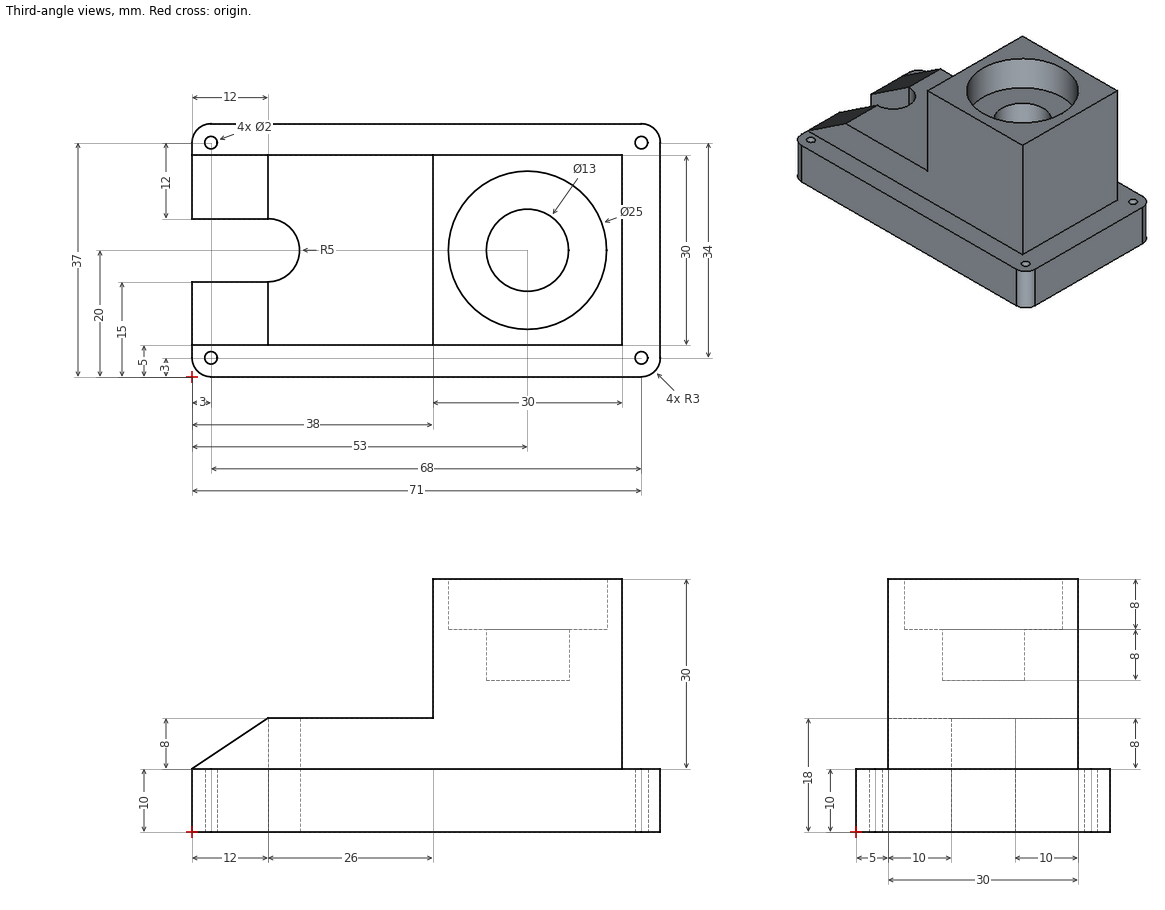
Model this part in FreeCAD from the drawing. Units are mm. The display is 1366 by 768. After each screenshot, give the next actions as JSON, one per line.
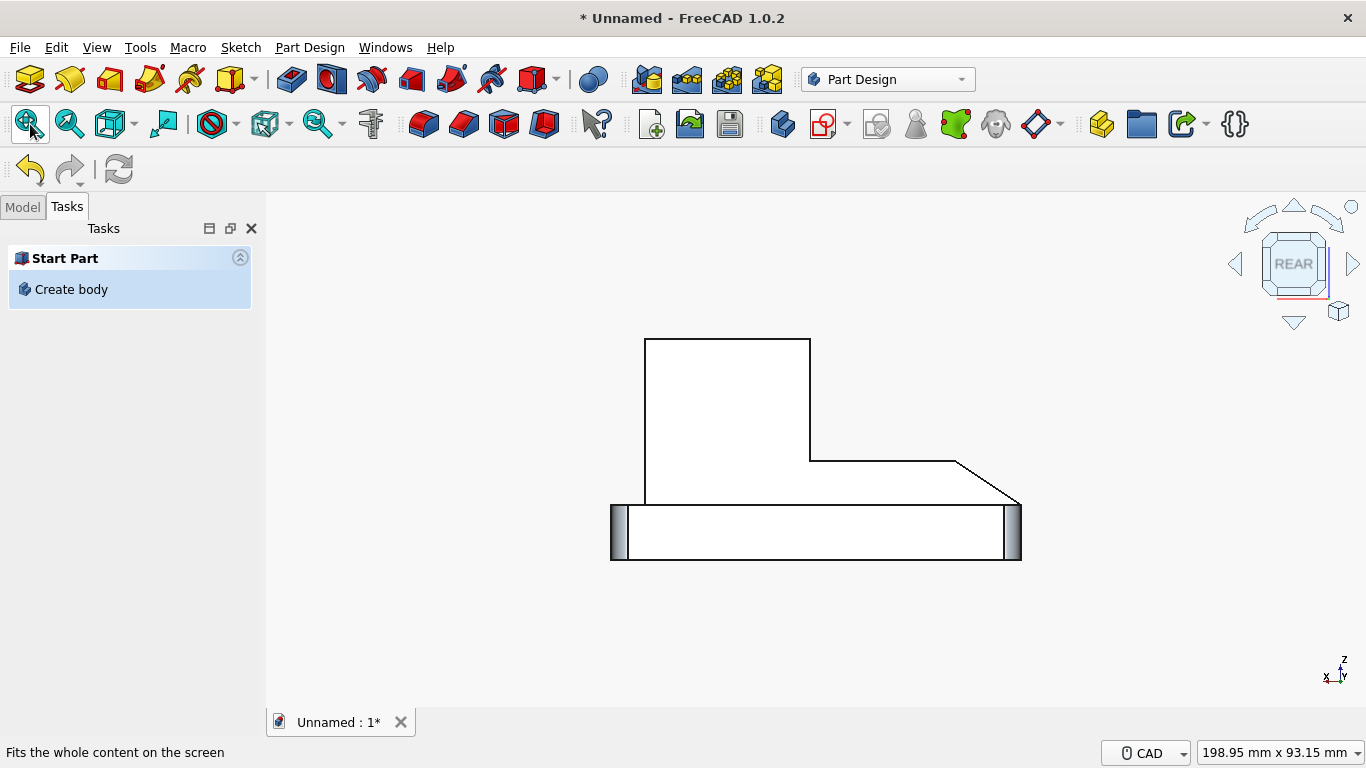
{"action": "key", "text": "0"}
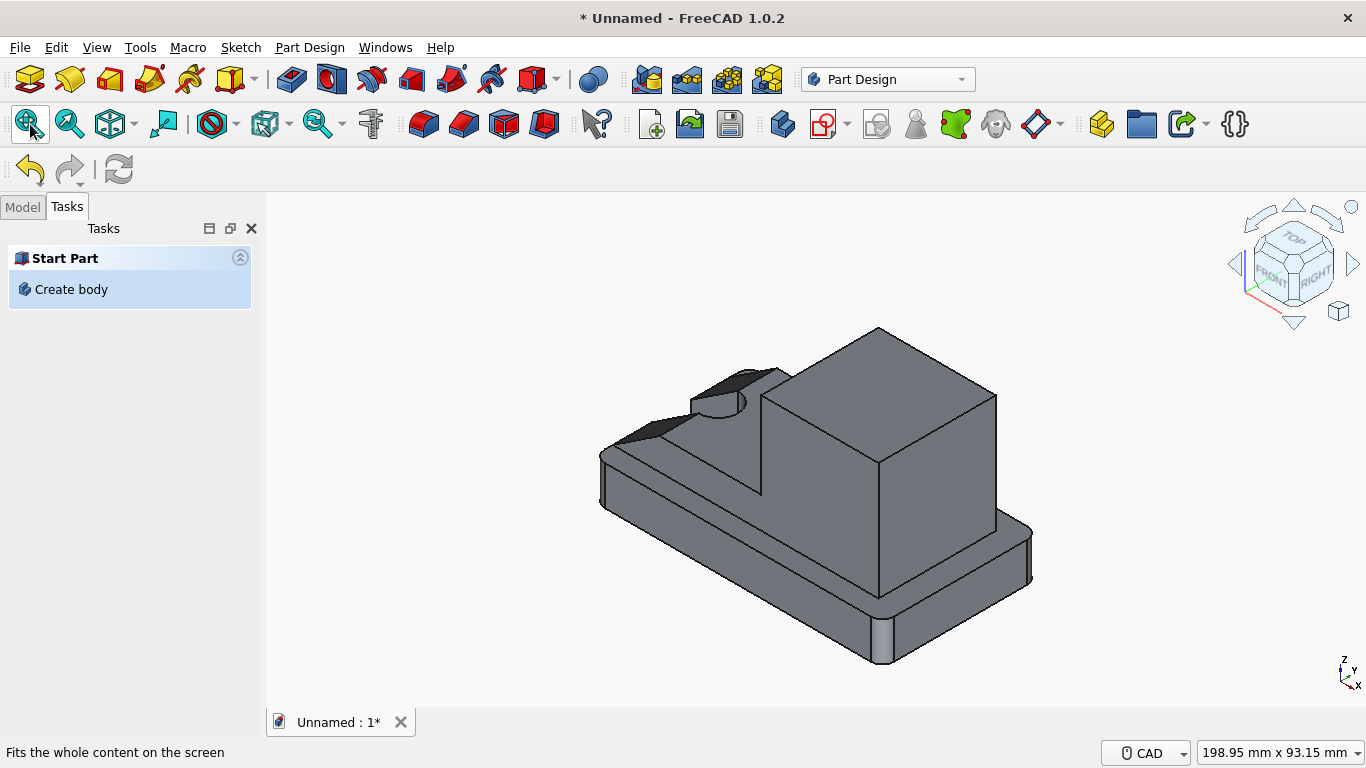
{"action": "left_click", "coordinate": [1007, 527]}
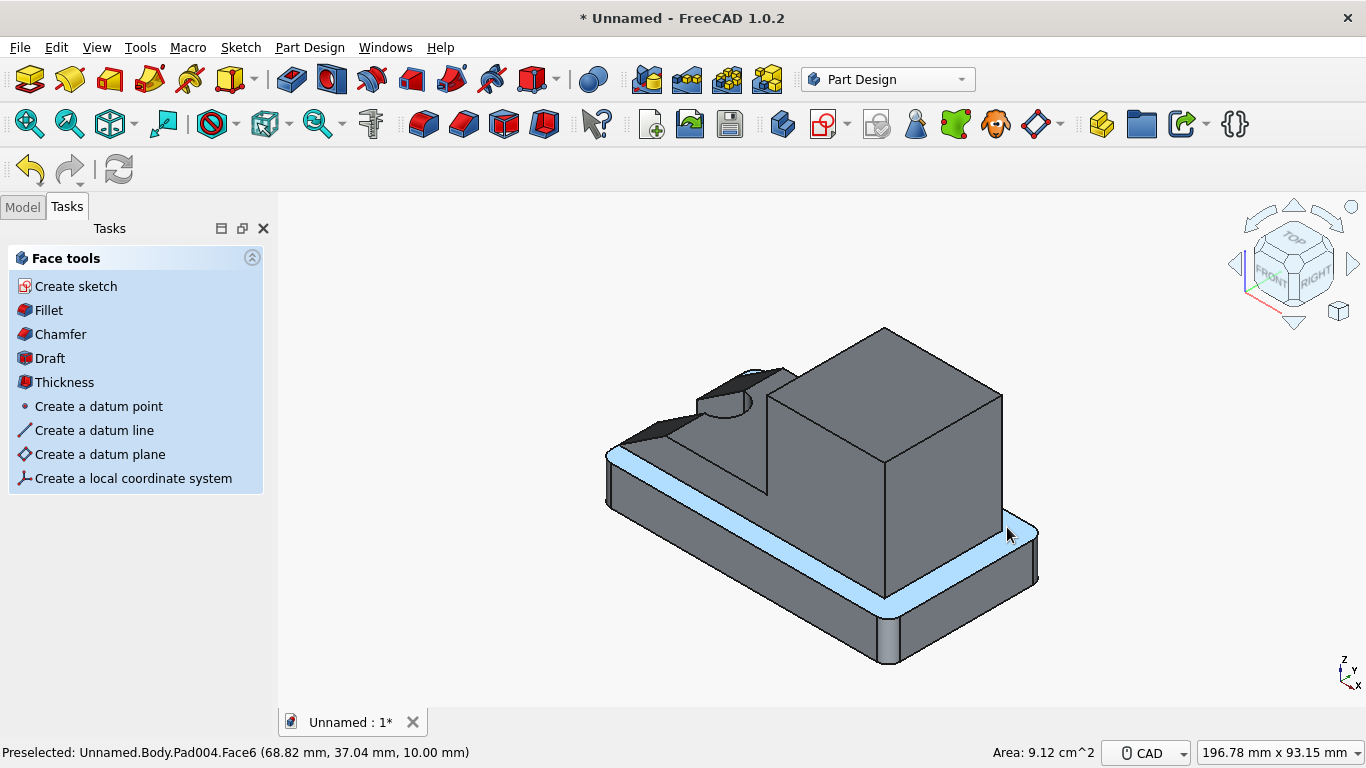
{"action": "left_click", "coordinate": [824, 124]}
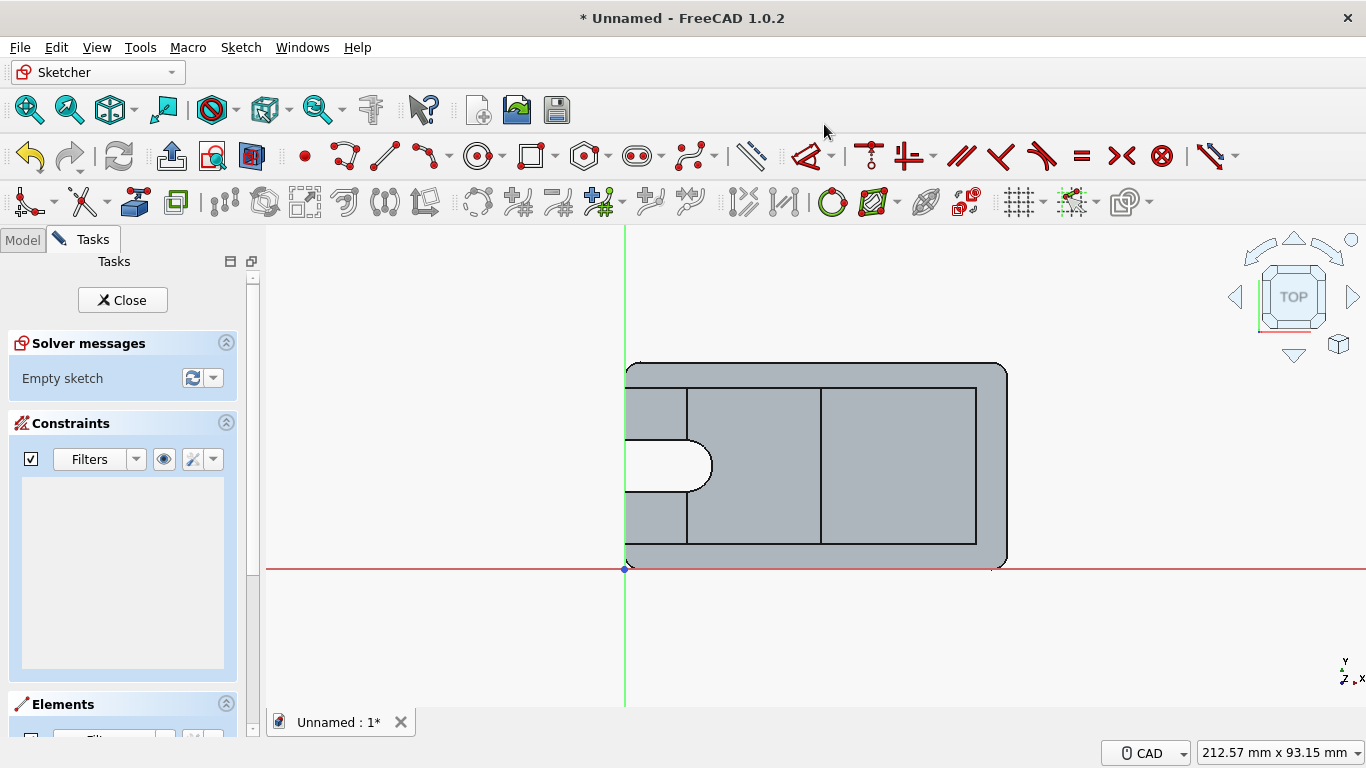
{"action": "scroll", "coordinate": [940, 482], "scroll_direction": "up", "scroll_amount": 2}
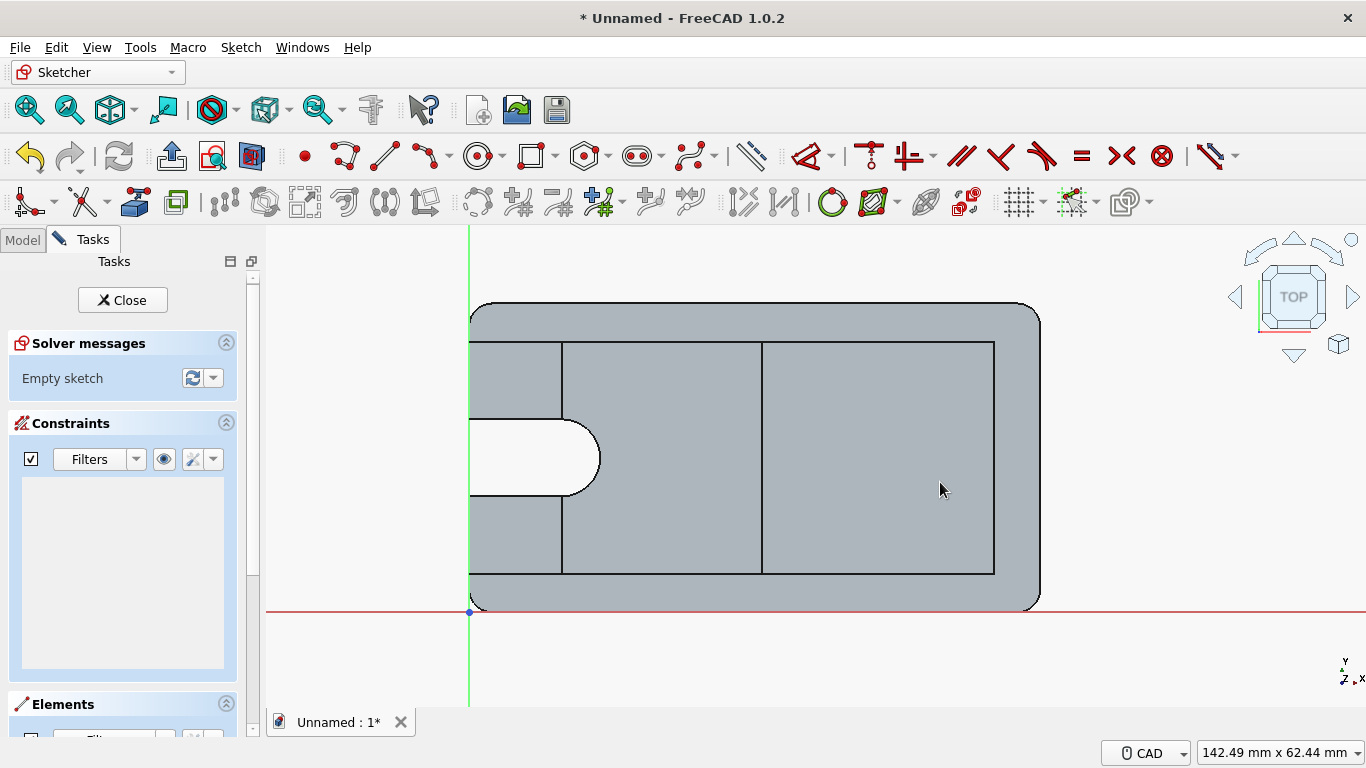
{"action": "left_click", "coordinate": [478, 156]}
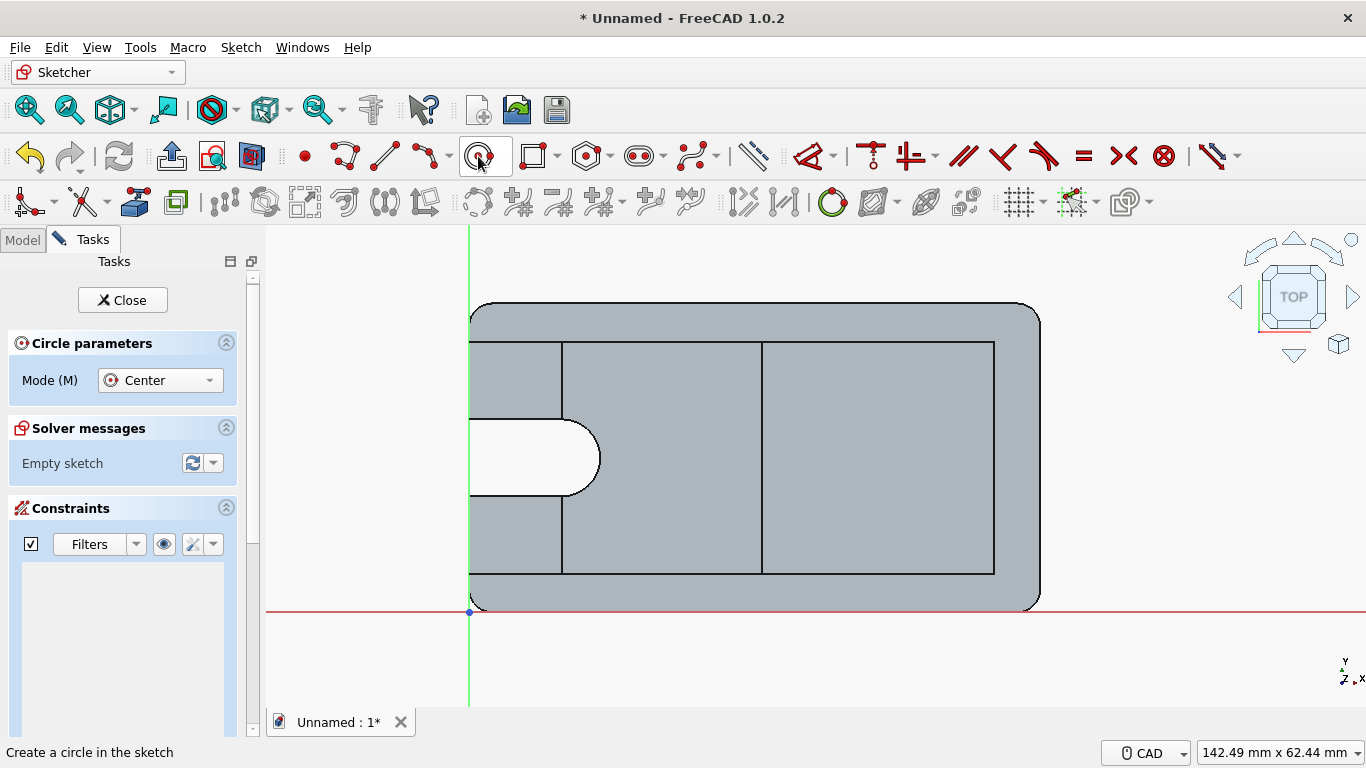
{"action": "scroll", "coordinate": [492, 327], "scroll_direction": "up", "scroll_amount": 6}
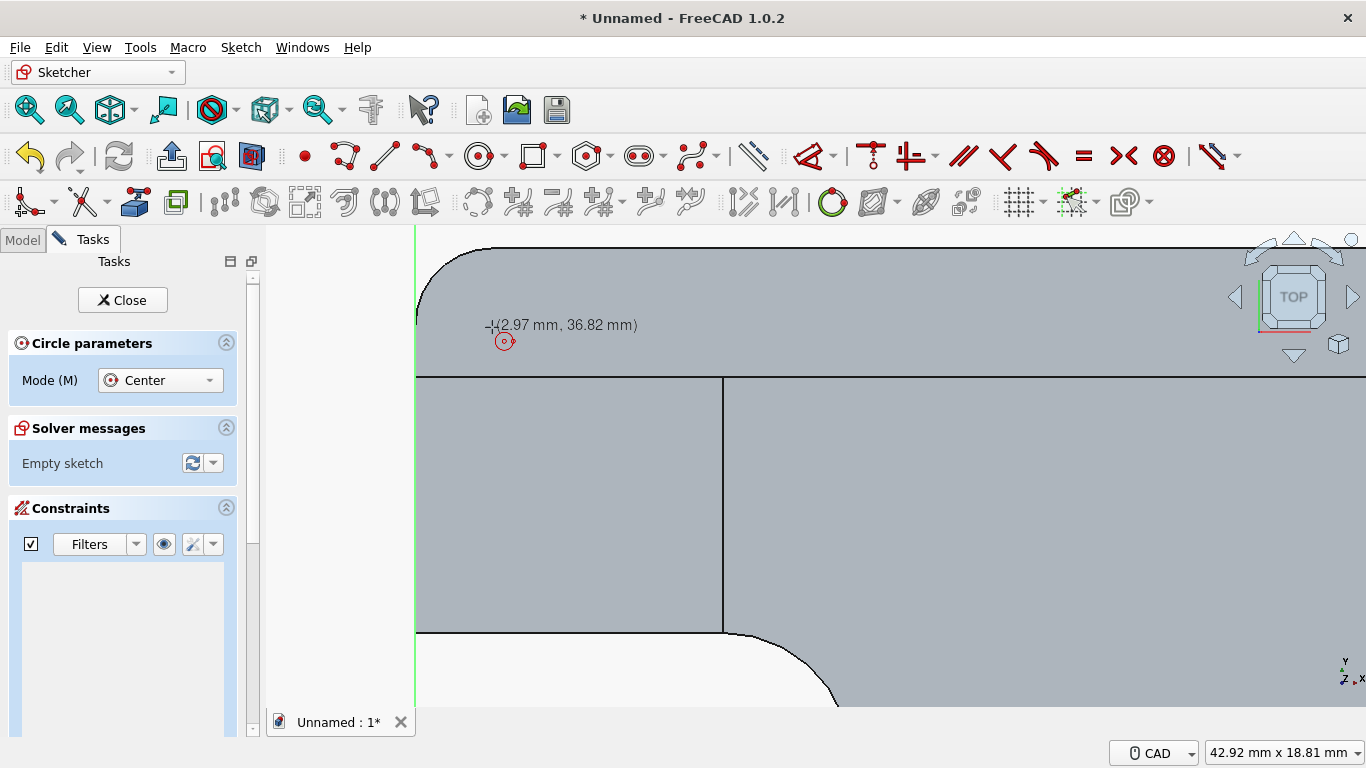
{"action": "left_click", "coordinate": [492, 325]}
{"action": "left_click", "coordinate": [510, 307]}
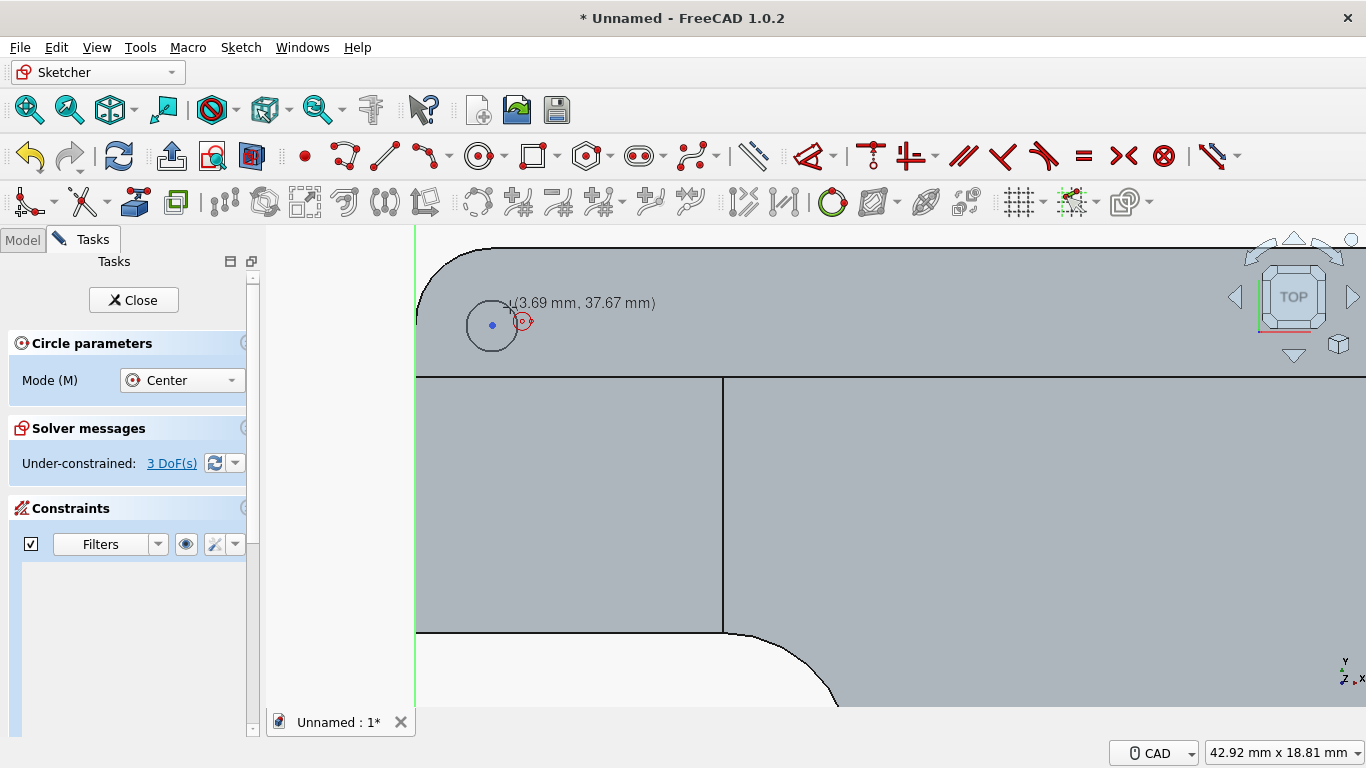
{"action": "scroll", "coordinate": [493, 328], "scroll_direction": "down", "scroll_amount": 6}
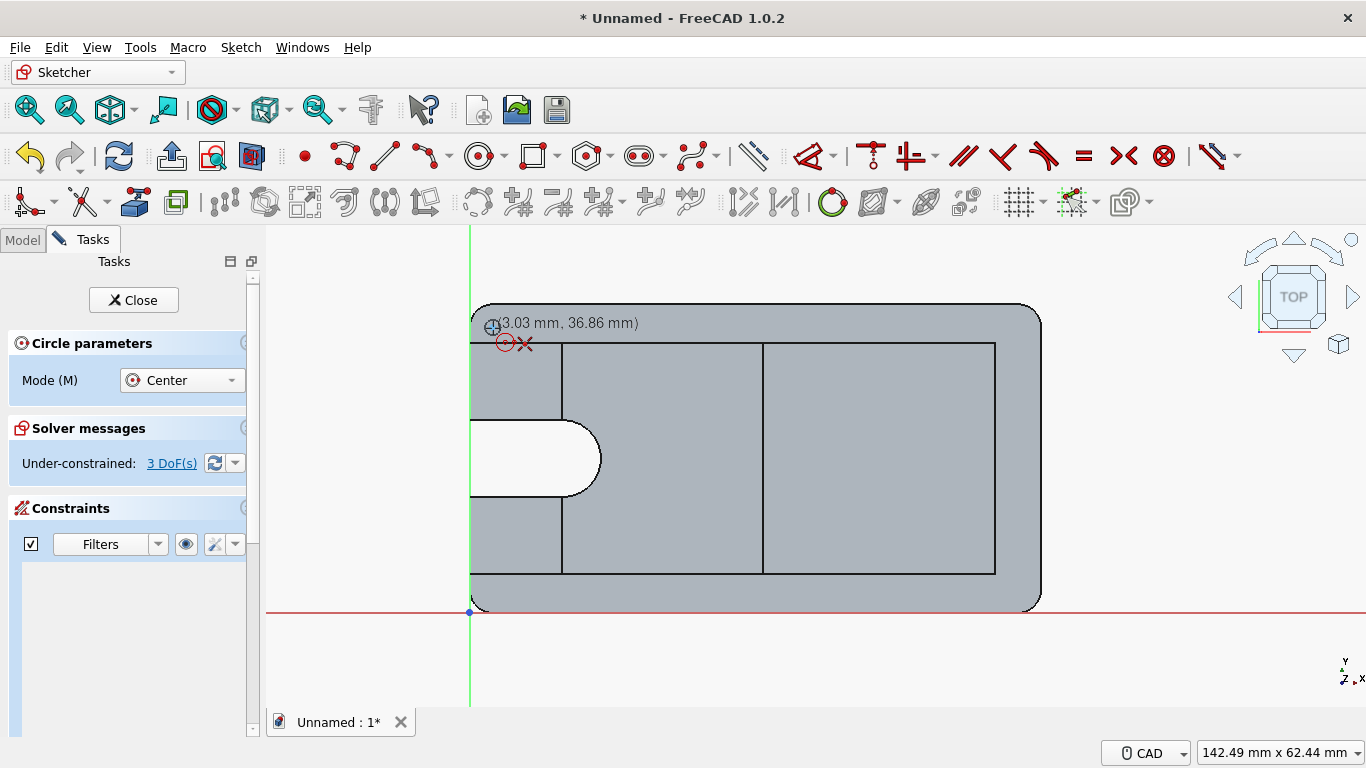
{"action": "scroll", "coordinate": [1018, 327], "scroll_direction": "up", "scroll_amount": 6}